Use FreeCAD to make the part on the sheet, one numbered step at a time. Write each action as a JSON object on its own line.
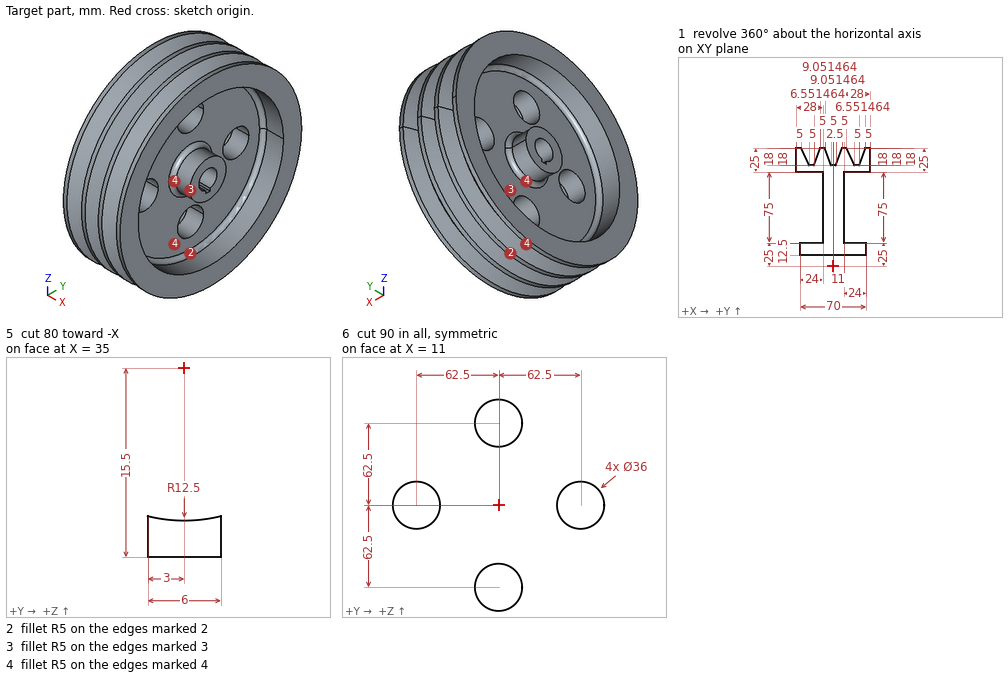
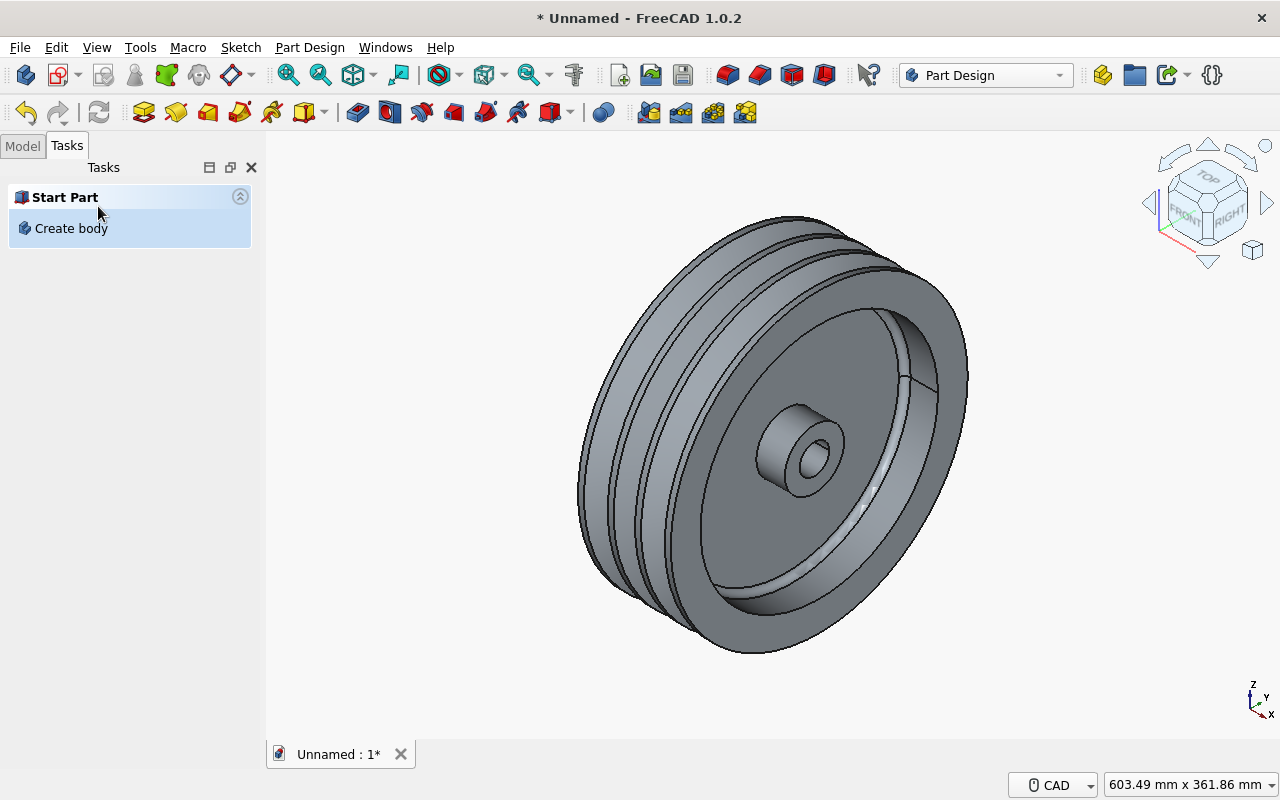
{"action": "key", "text": "1"}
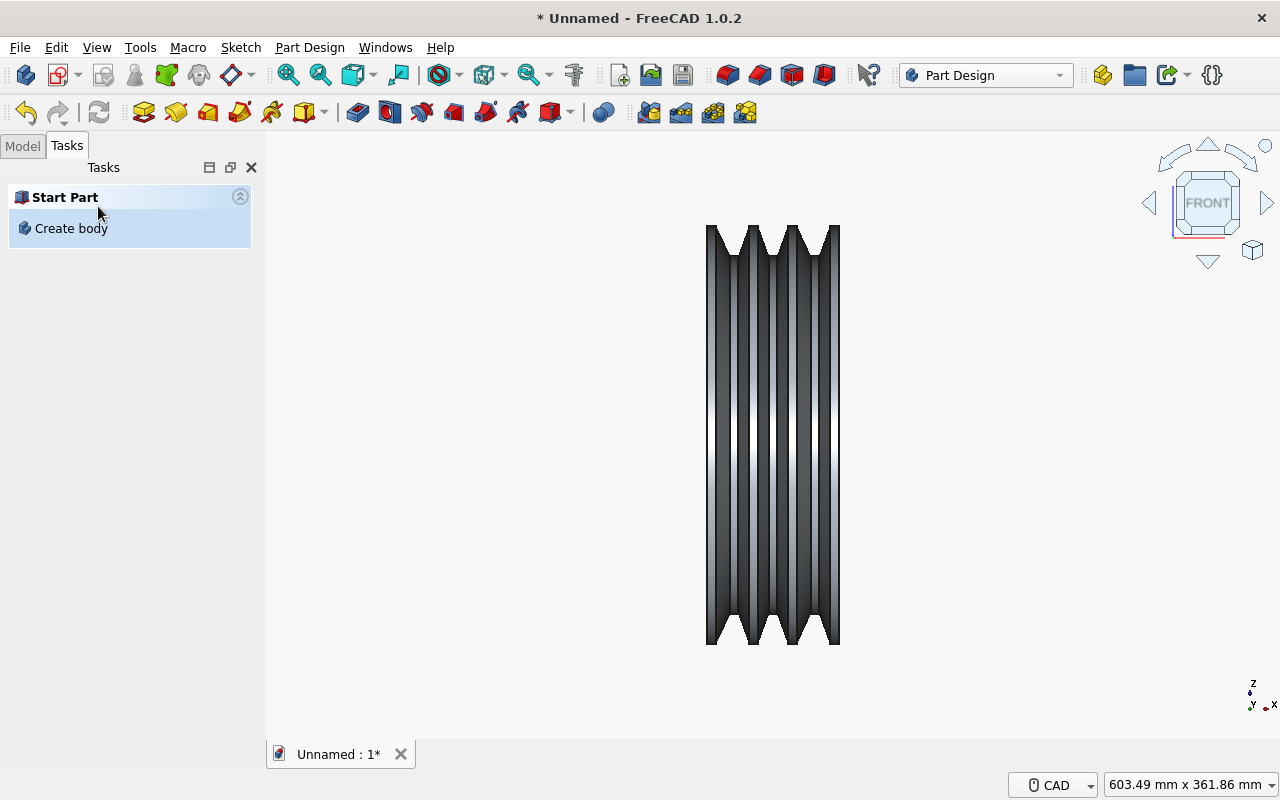
{"action": "key", "text": "3"}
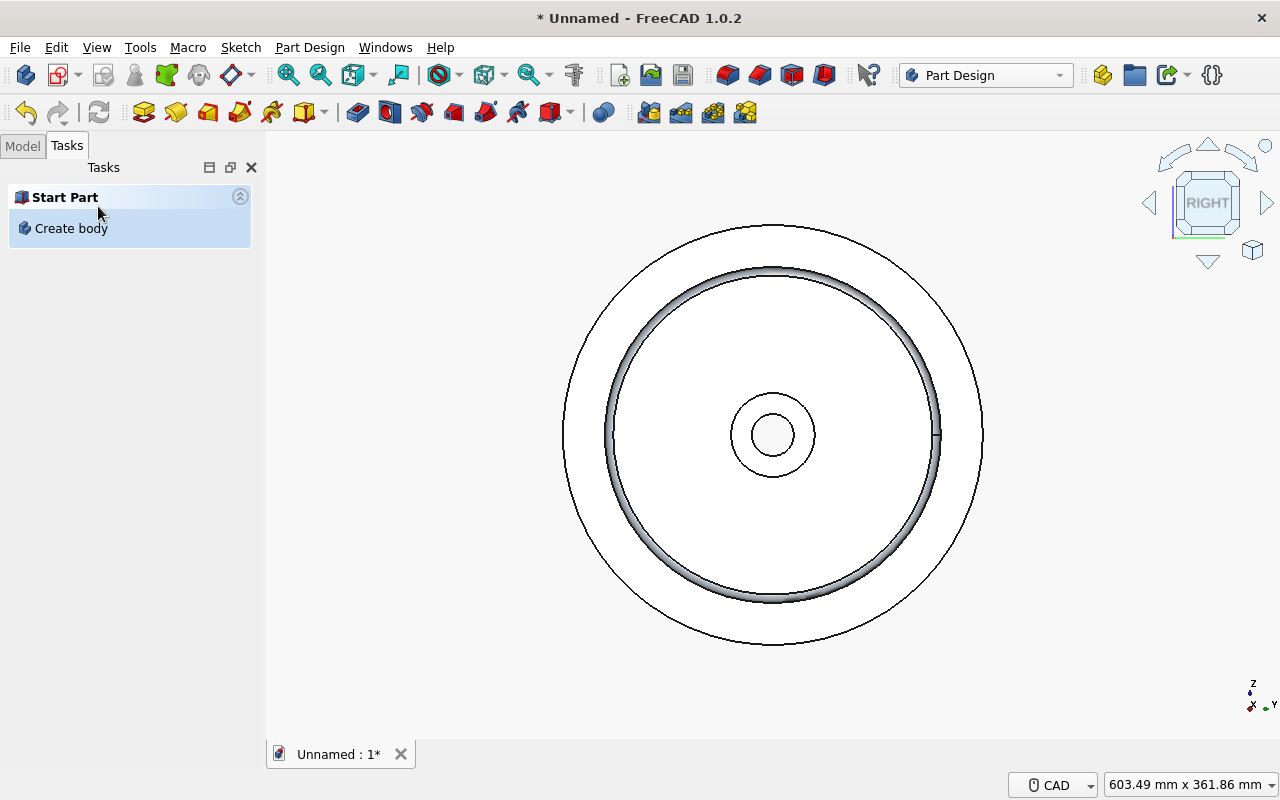
{"action": "key", "text": "5"}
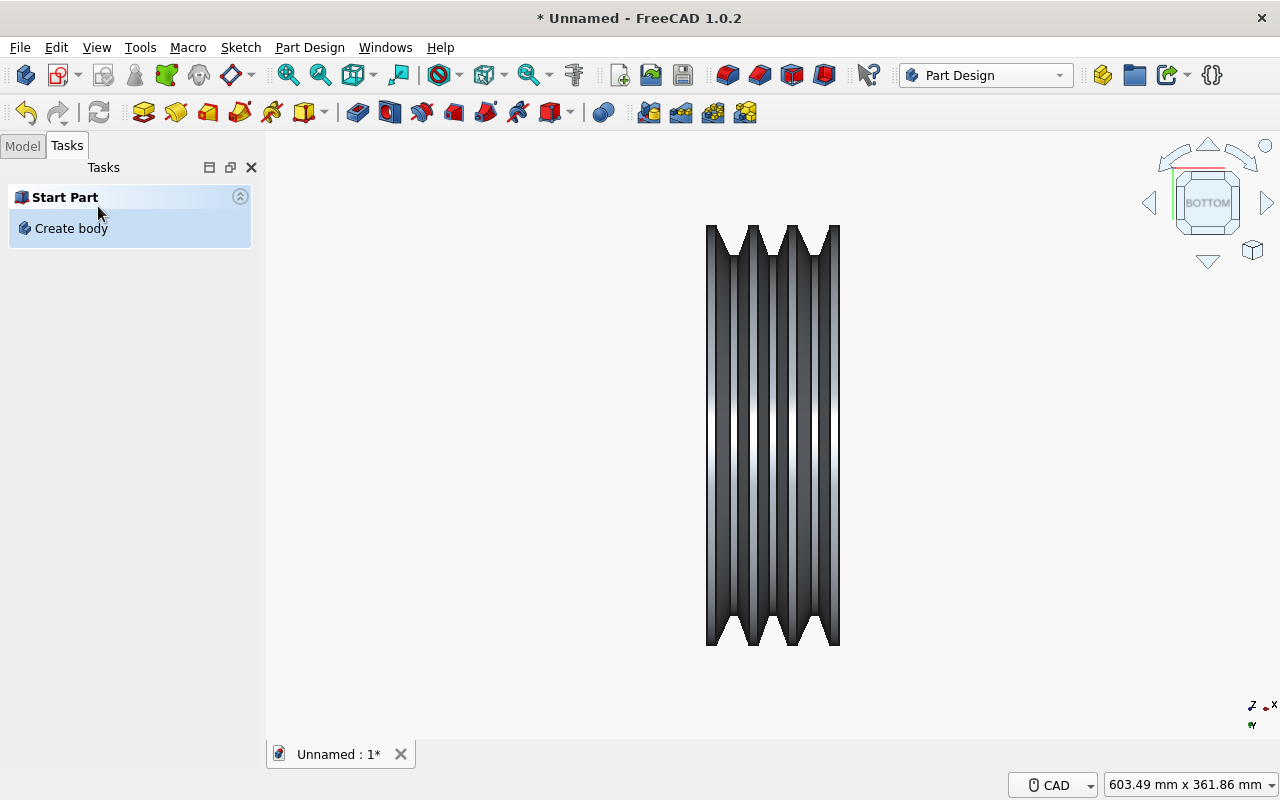
{"action": "key", "text": "4"}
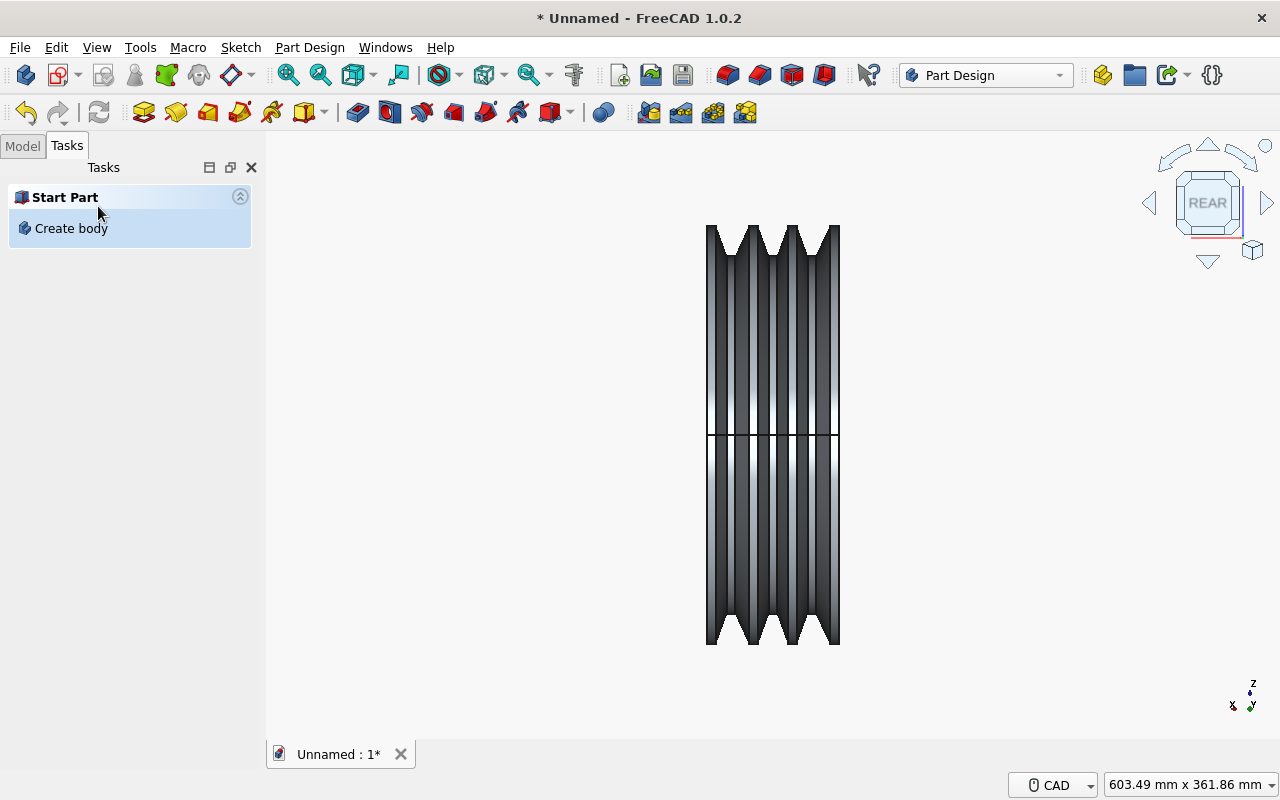
{"action": "key", "text": "6"}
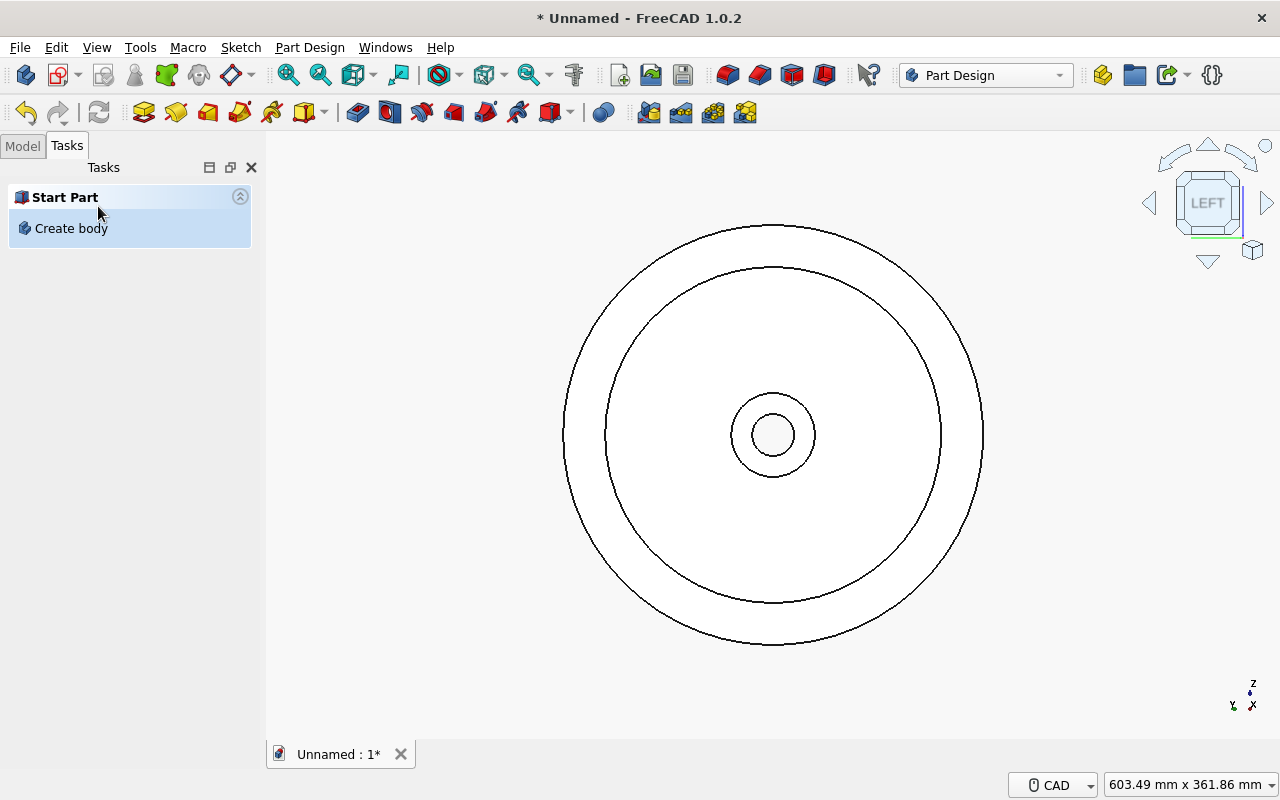
{"action": "key", "text": "v 3"}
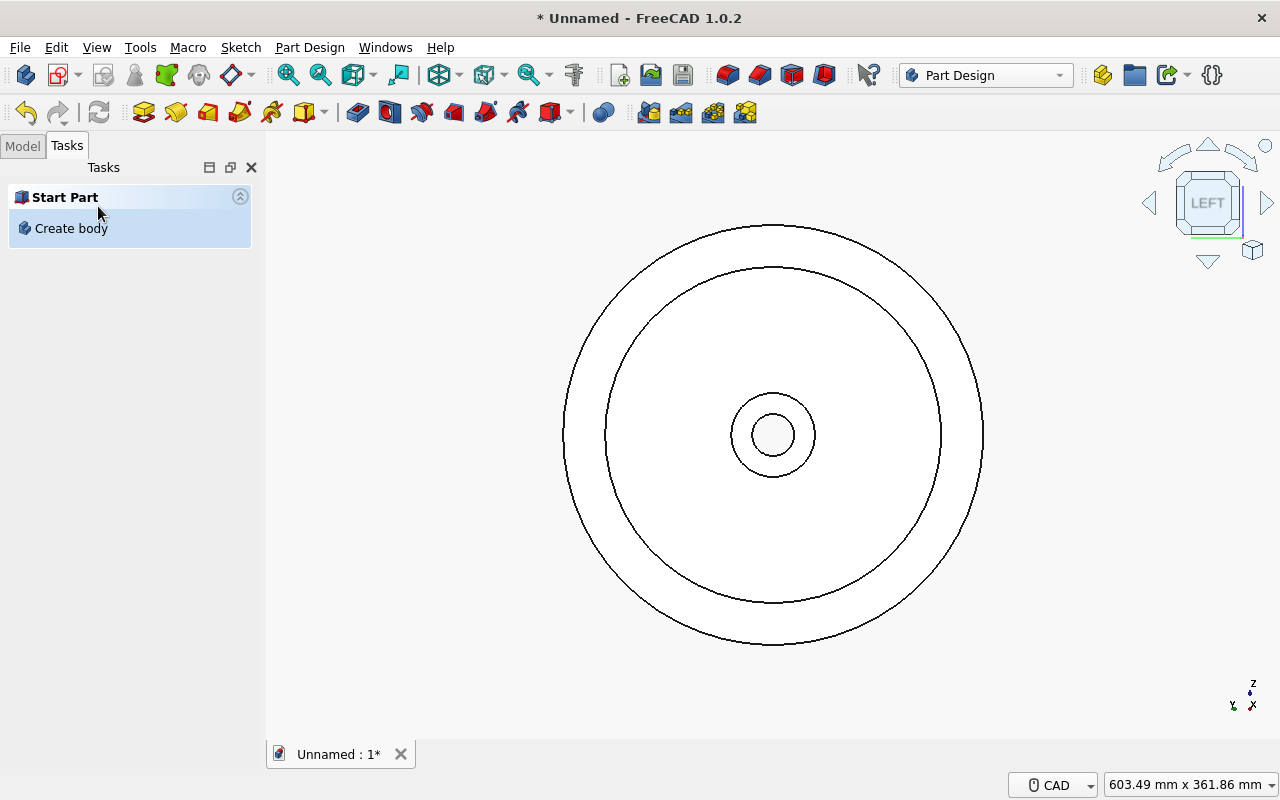
{"action": "key", "text": "0"}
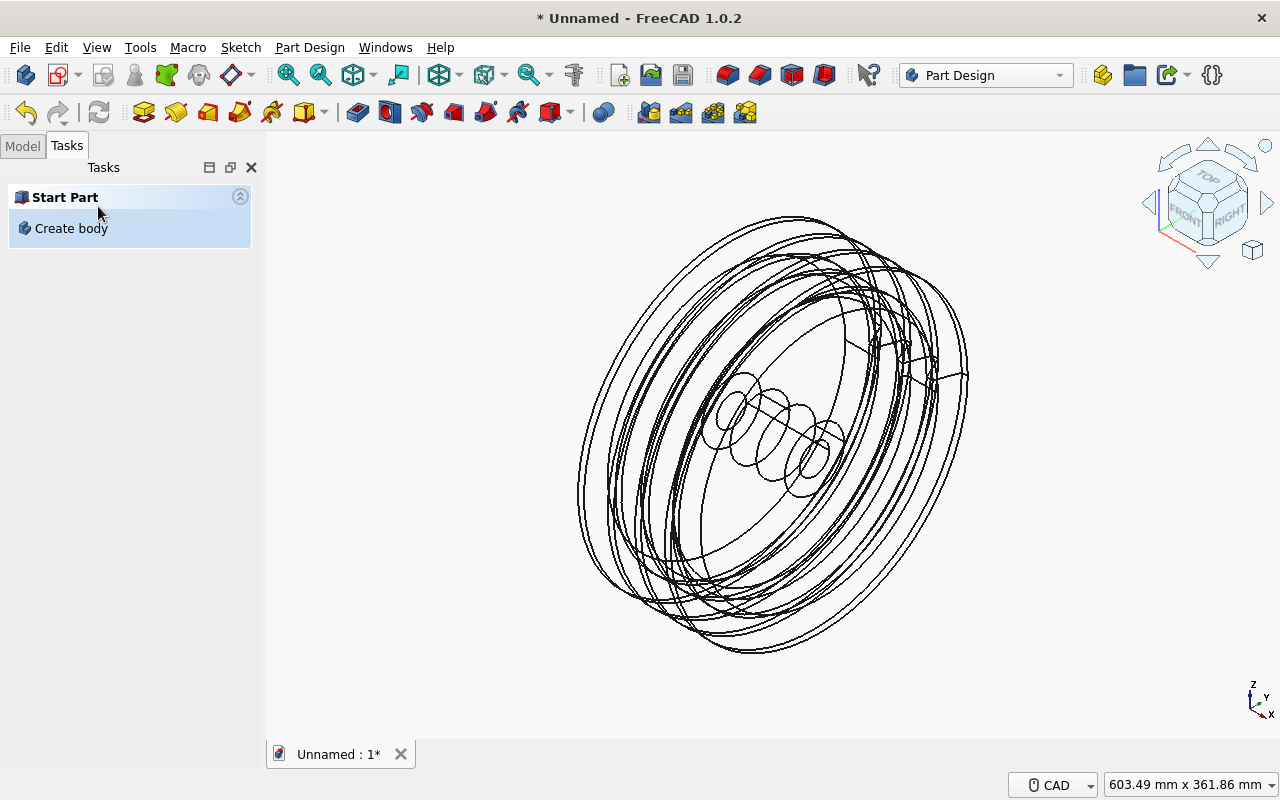
{"action": "left_click", "coordinate": [756, 459]}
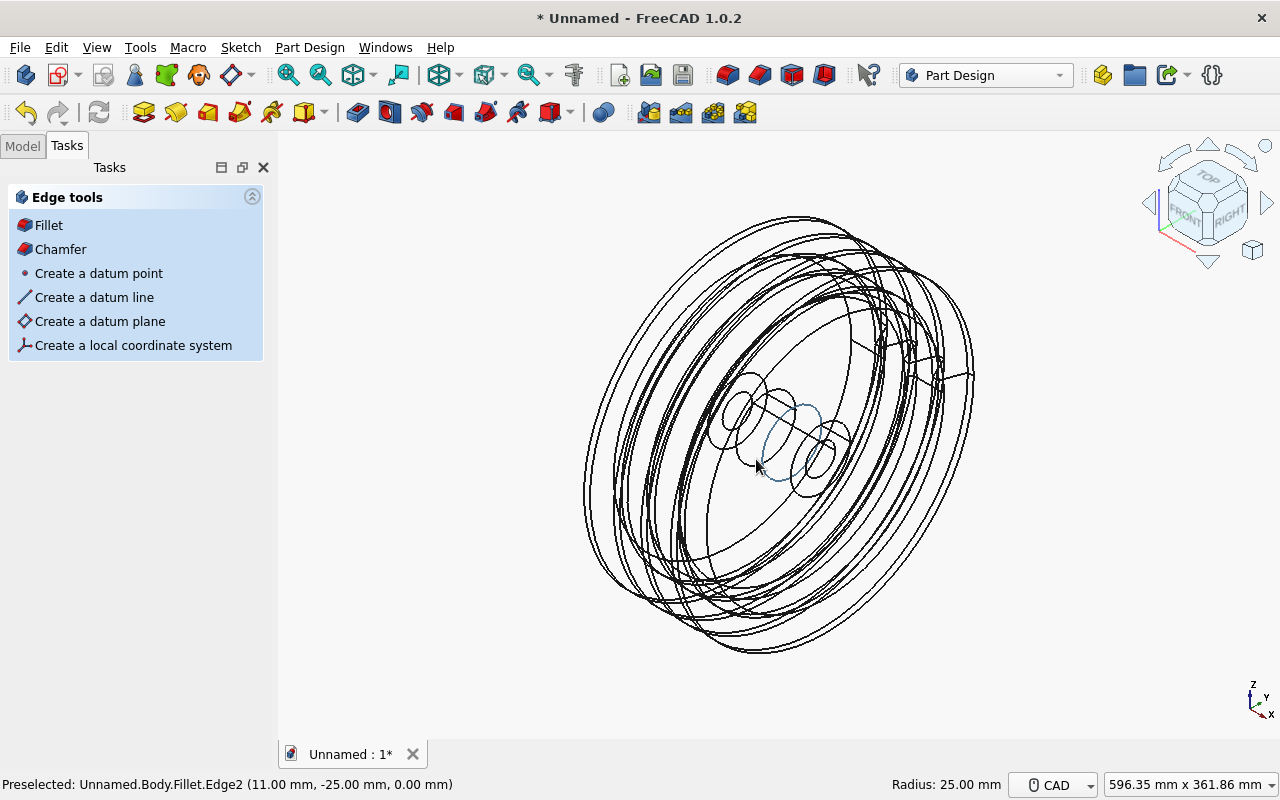
{"action": "key", "text": "v 1"}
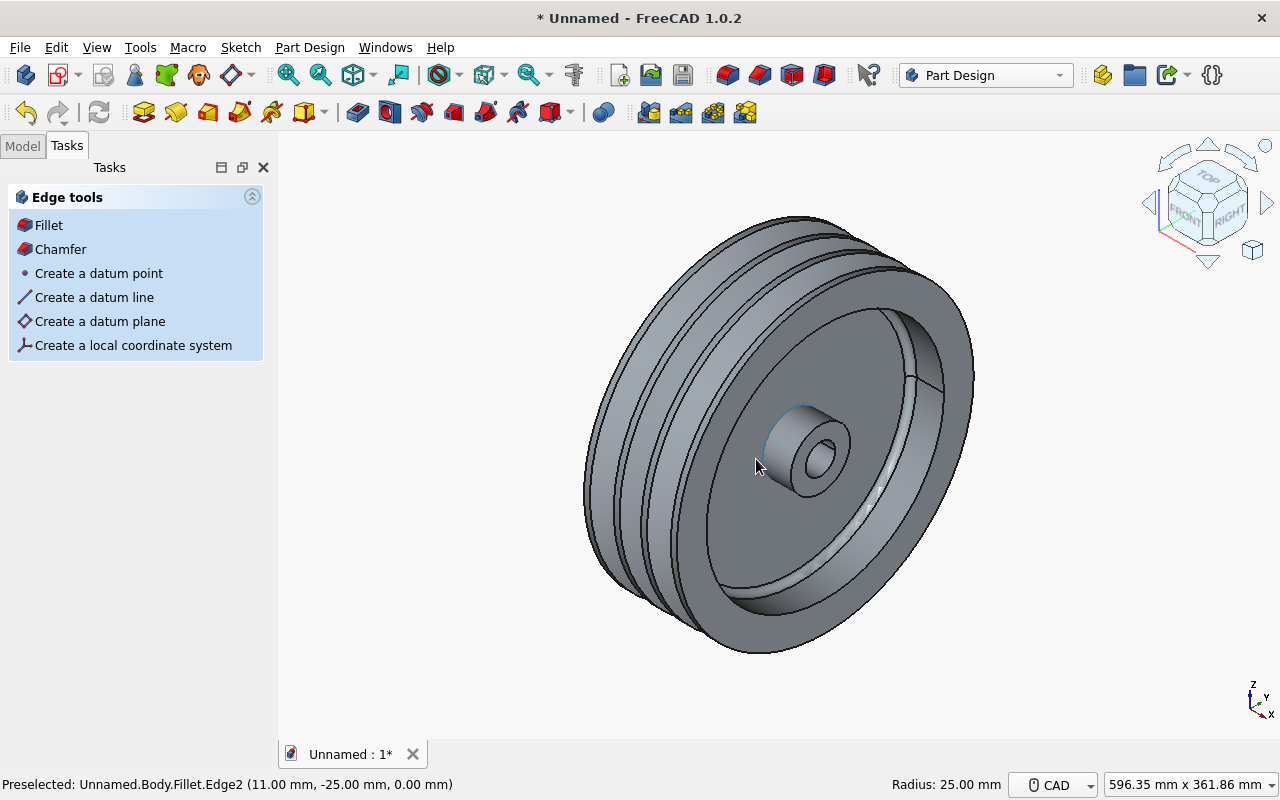
{"action": "left_click", "coordinate": [728, 76]}